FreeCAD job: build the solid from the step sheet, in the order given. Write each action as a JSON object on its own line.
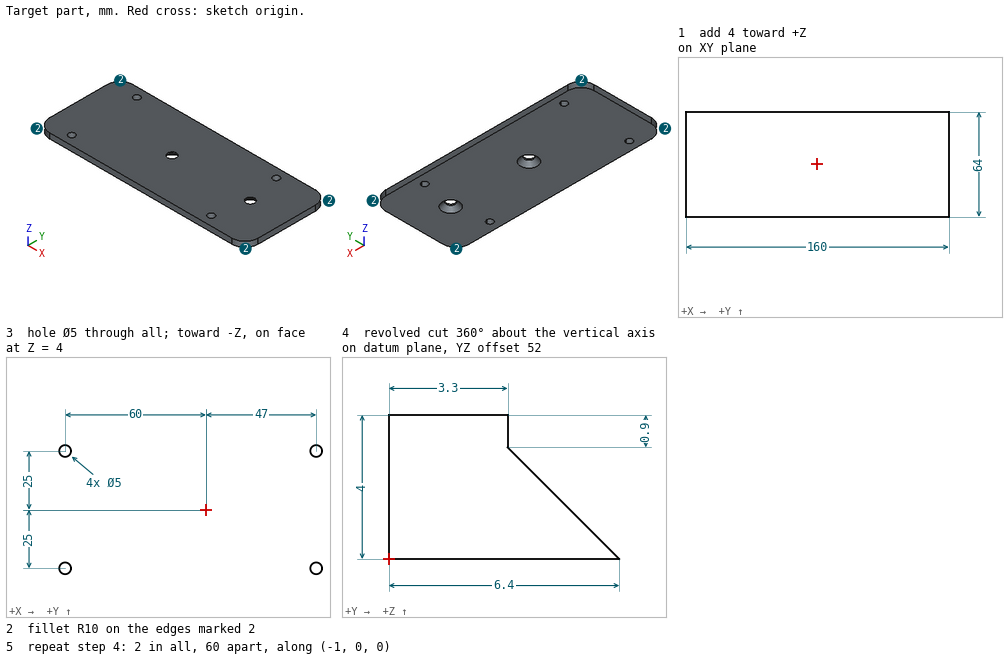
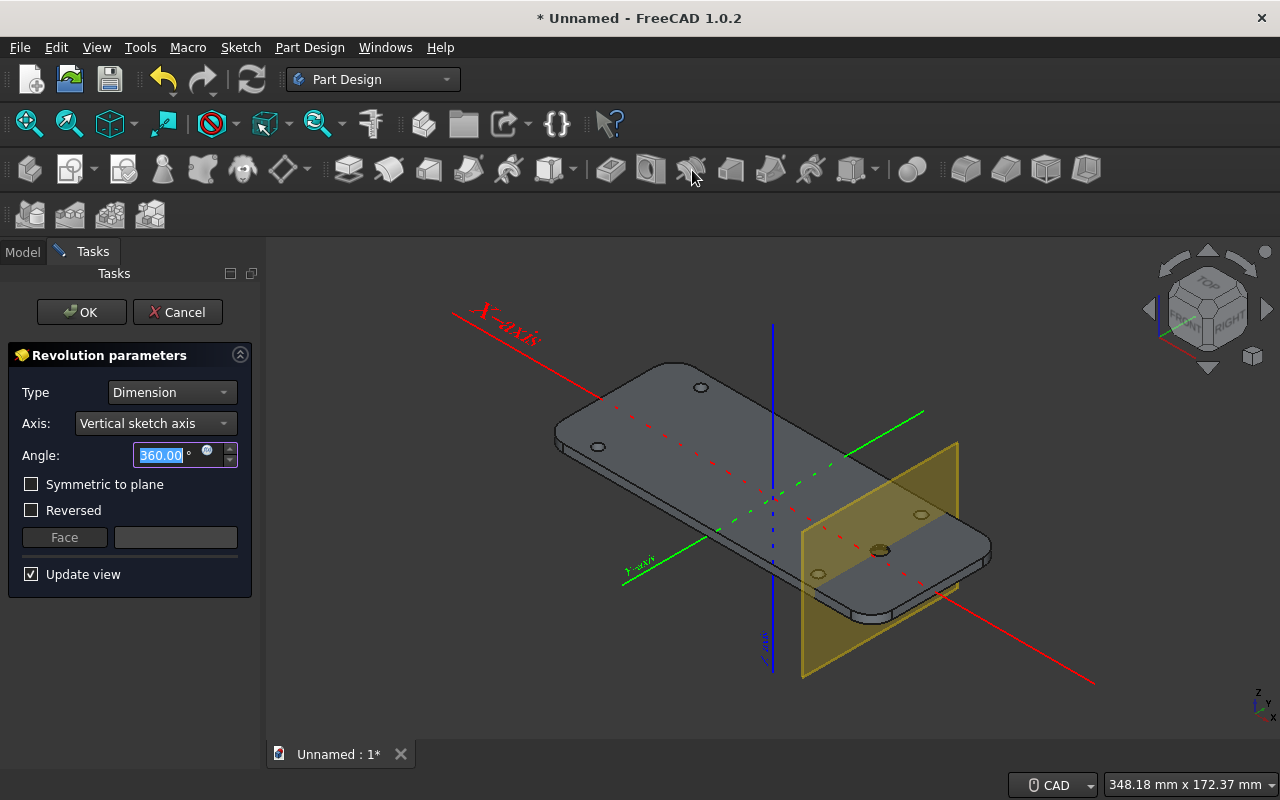
{"action": "left_click", "coordinate": [82, 312]}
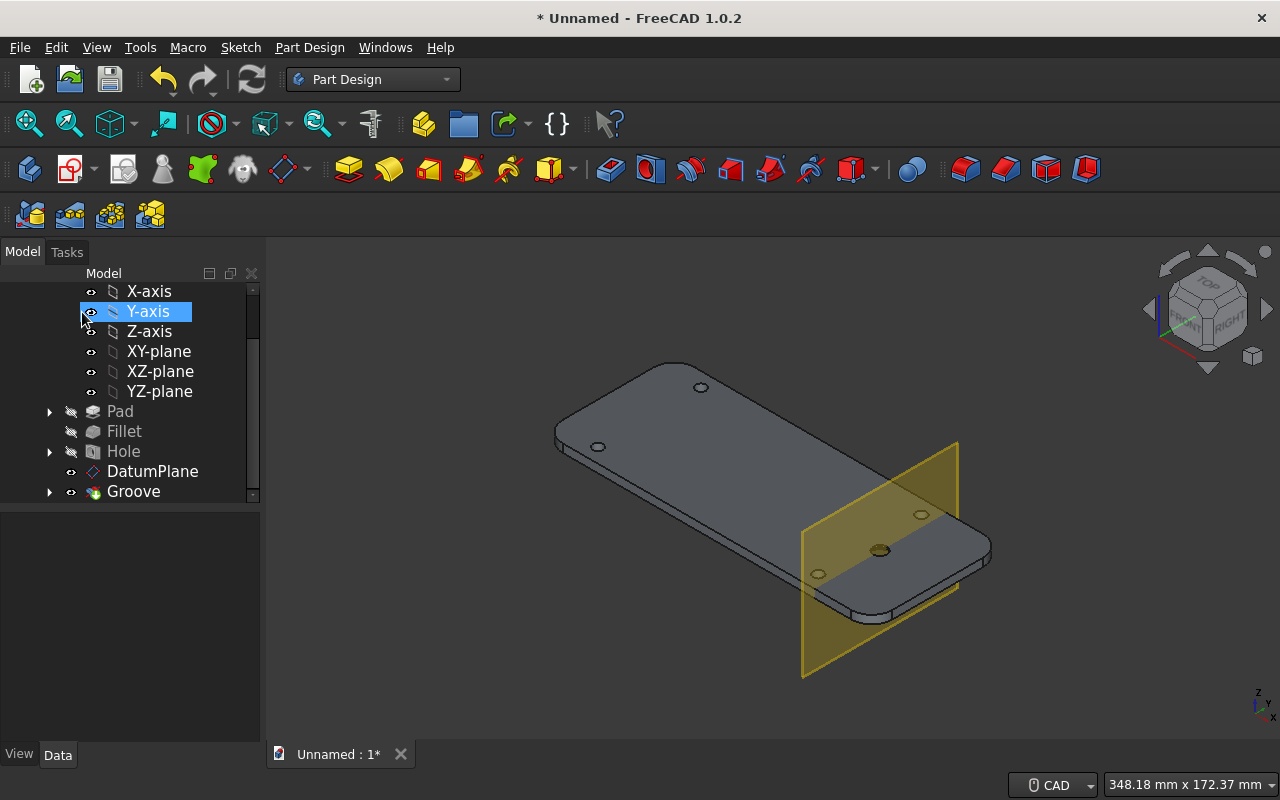
{"action": "left_click", "coordinate": [116, 472]}
{"action": "key", "text": "space"}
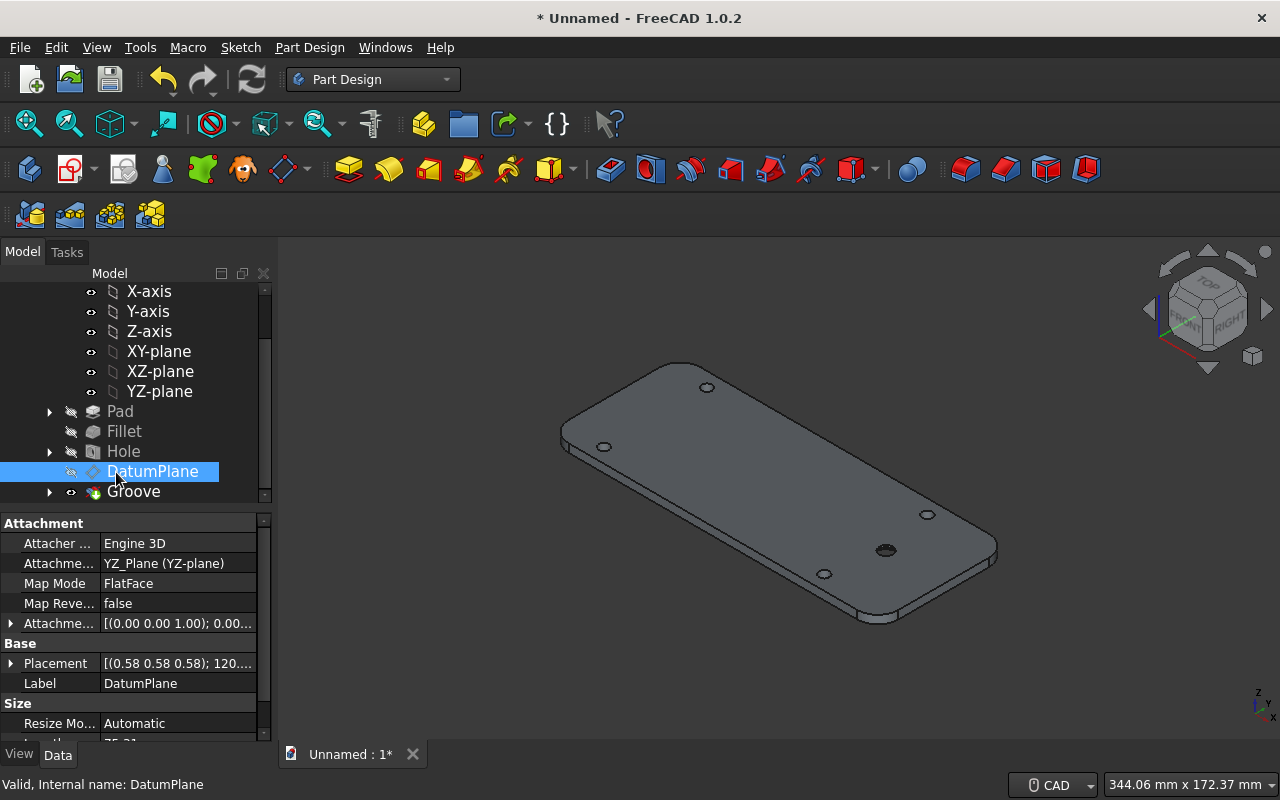
{"action": "left_click", "coordinate": [116, 492]}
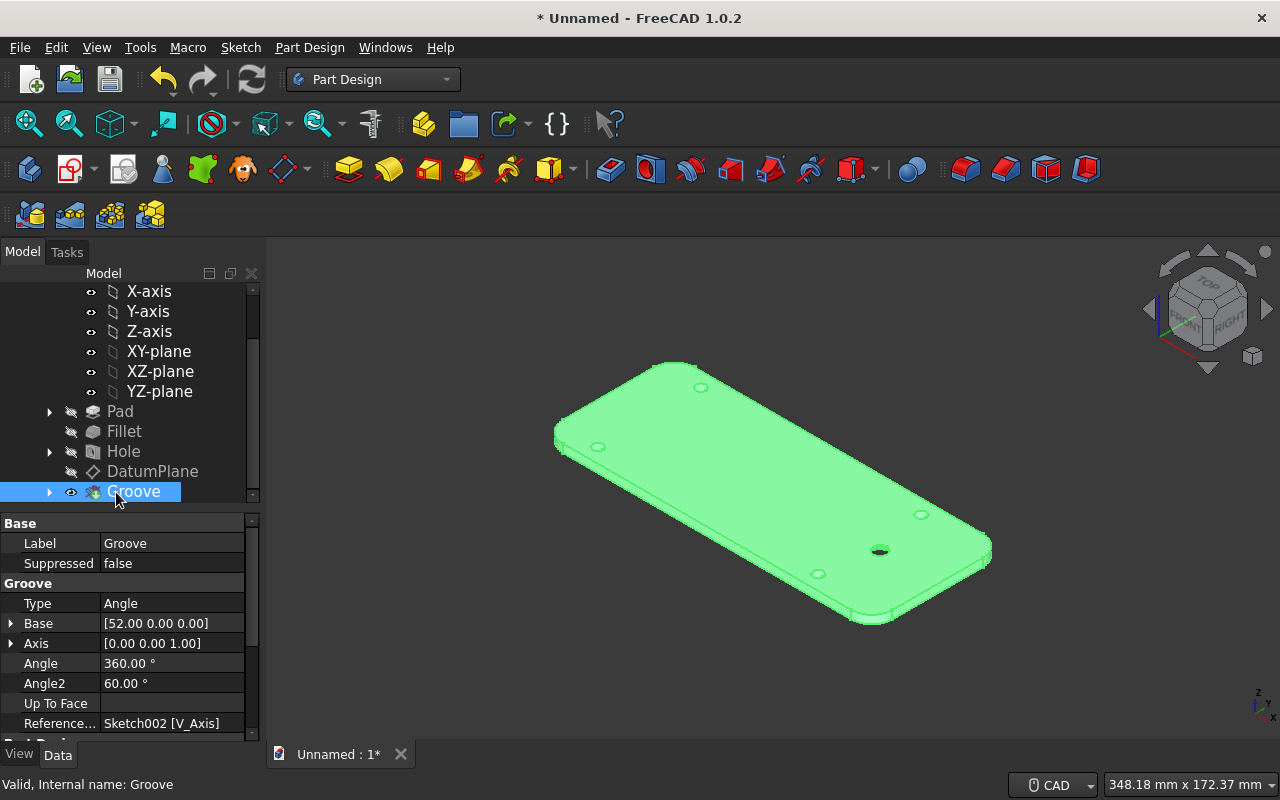
{"action": "left_click", "coordinate": [70, 214]}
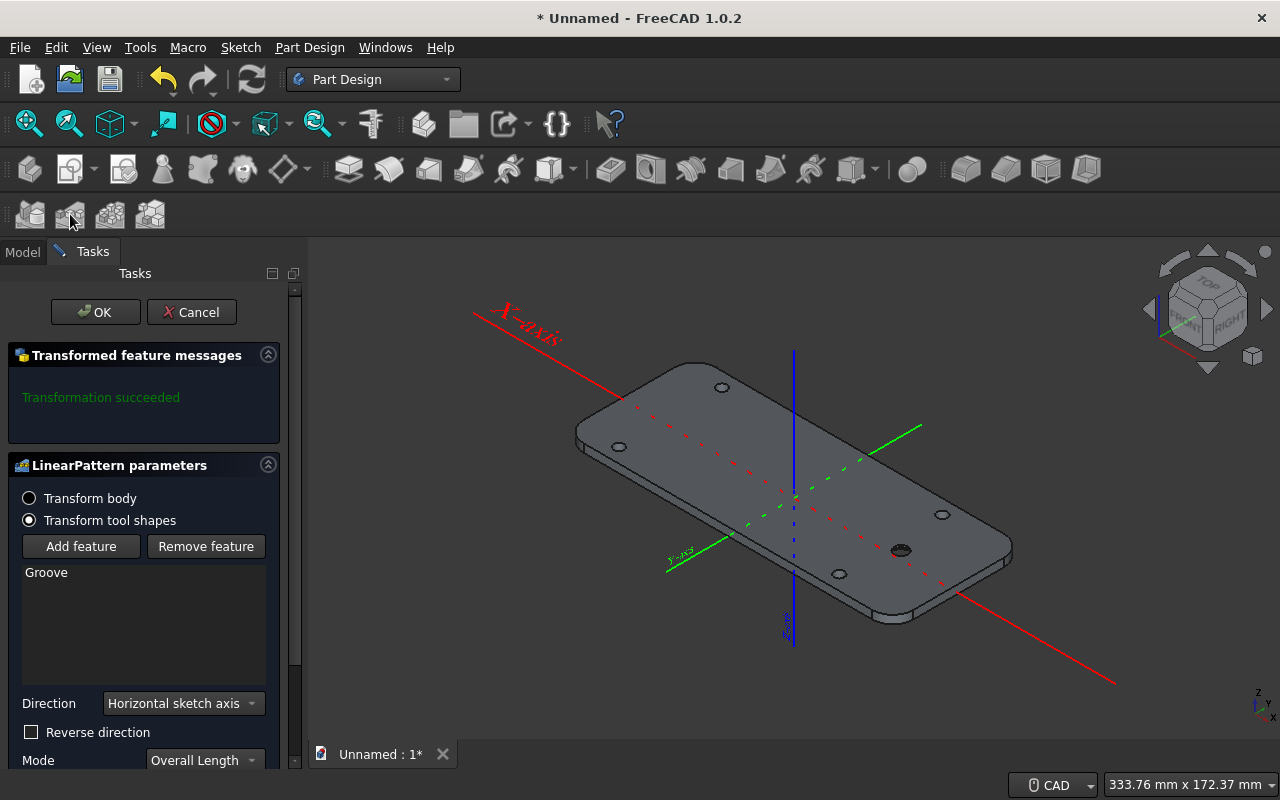
{"action": "left_click", "coordinate": [184, 704]}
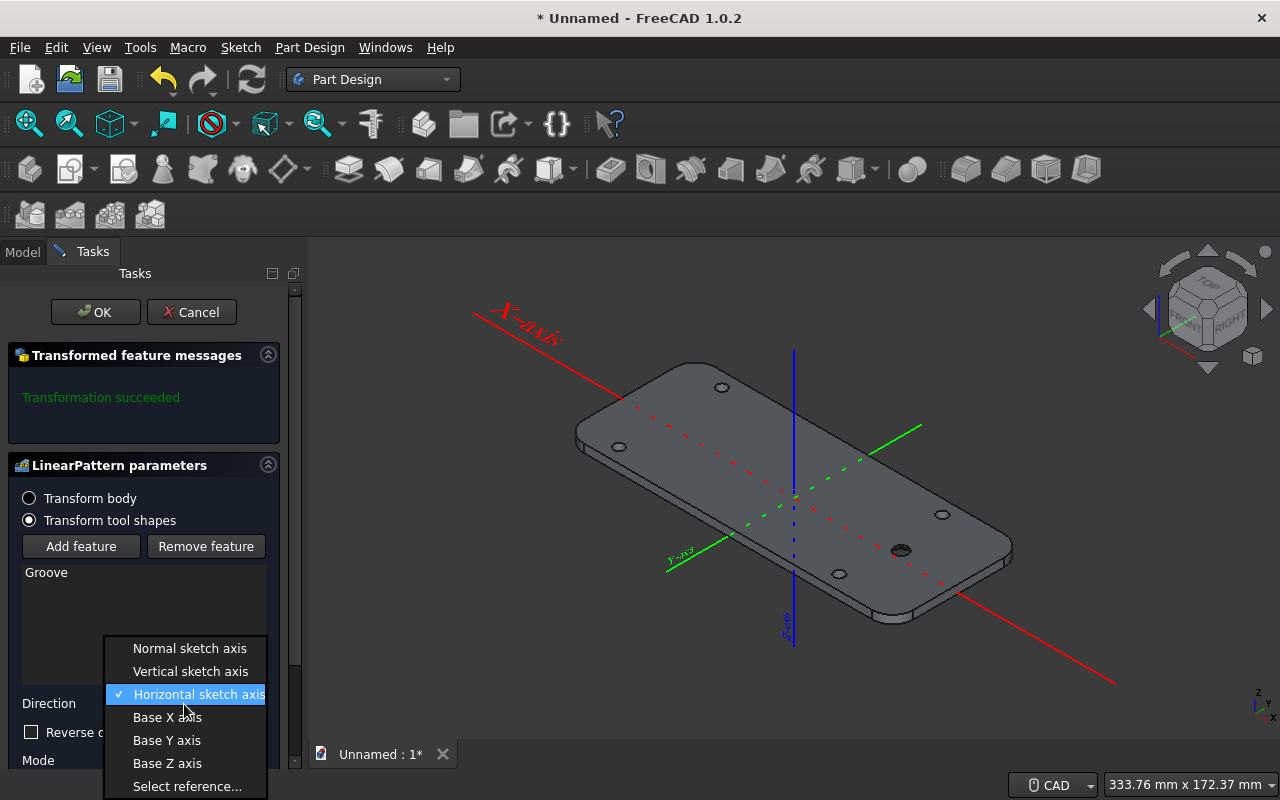
{"action": "left_click", "coordinate": [184, 718]}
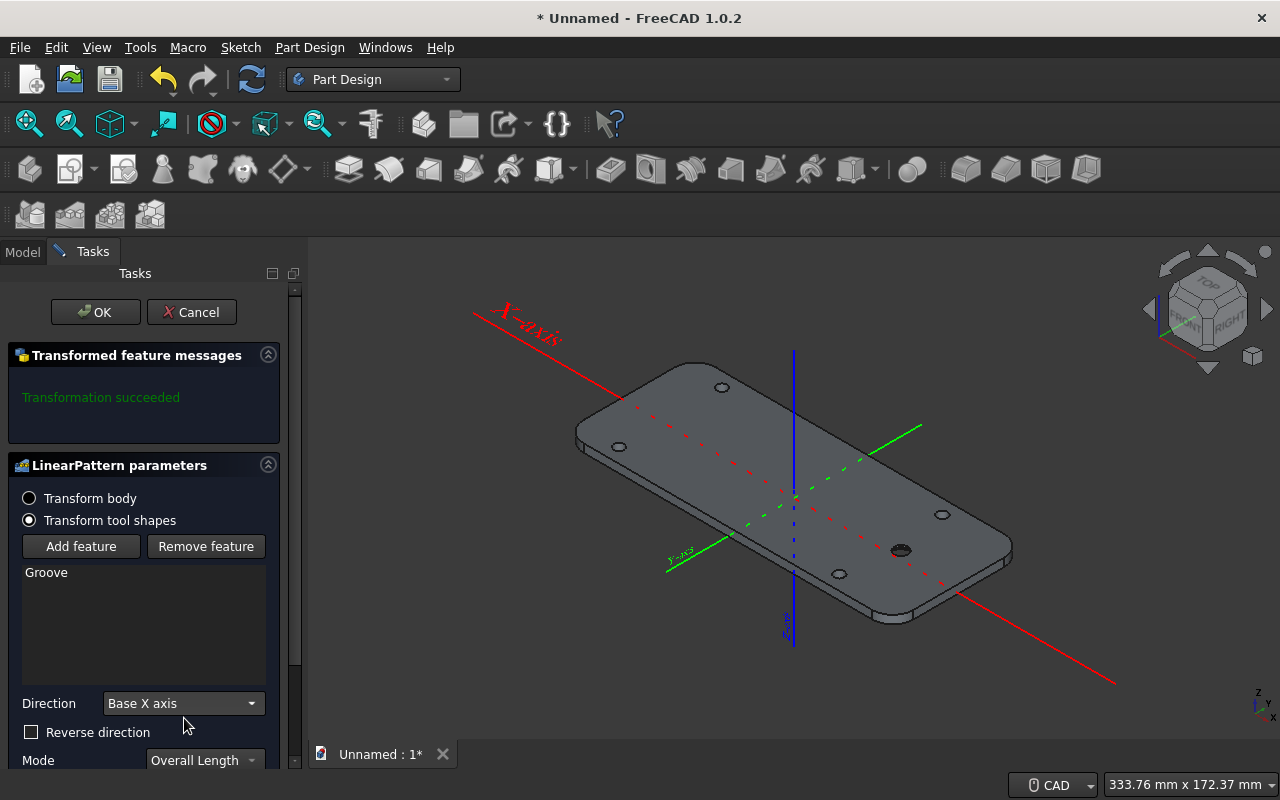
{"action": "scroll", "coordinate": [295, 526], "scroll_direction": "down", "scroll_amount": 2}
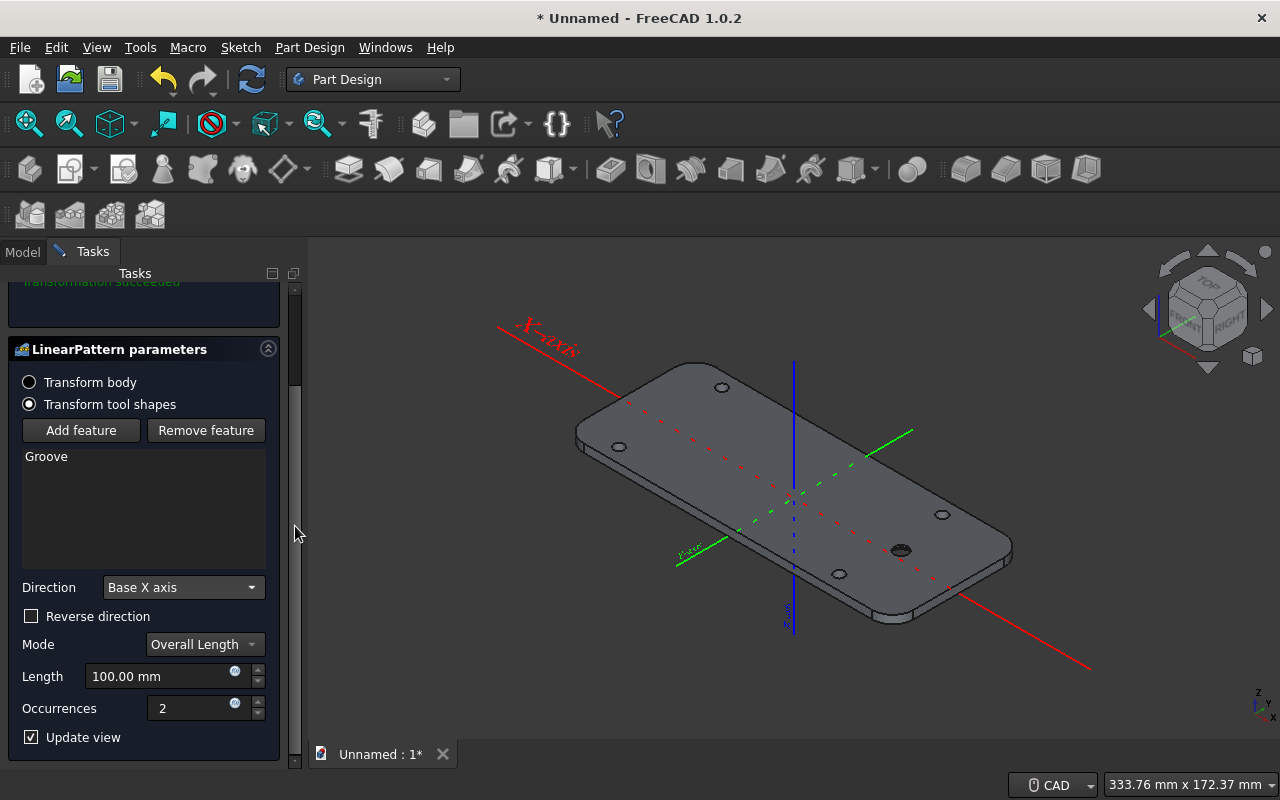
{"action": "left_click", "coordinate": [206, 644]}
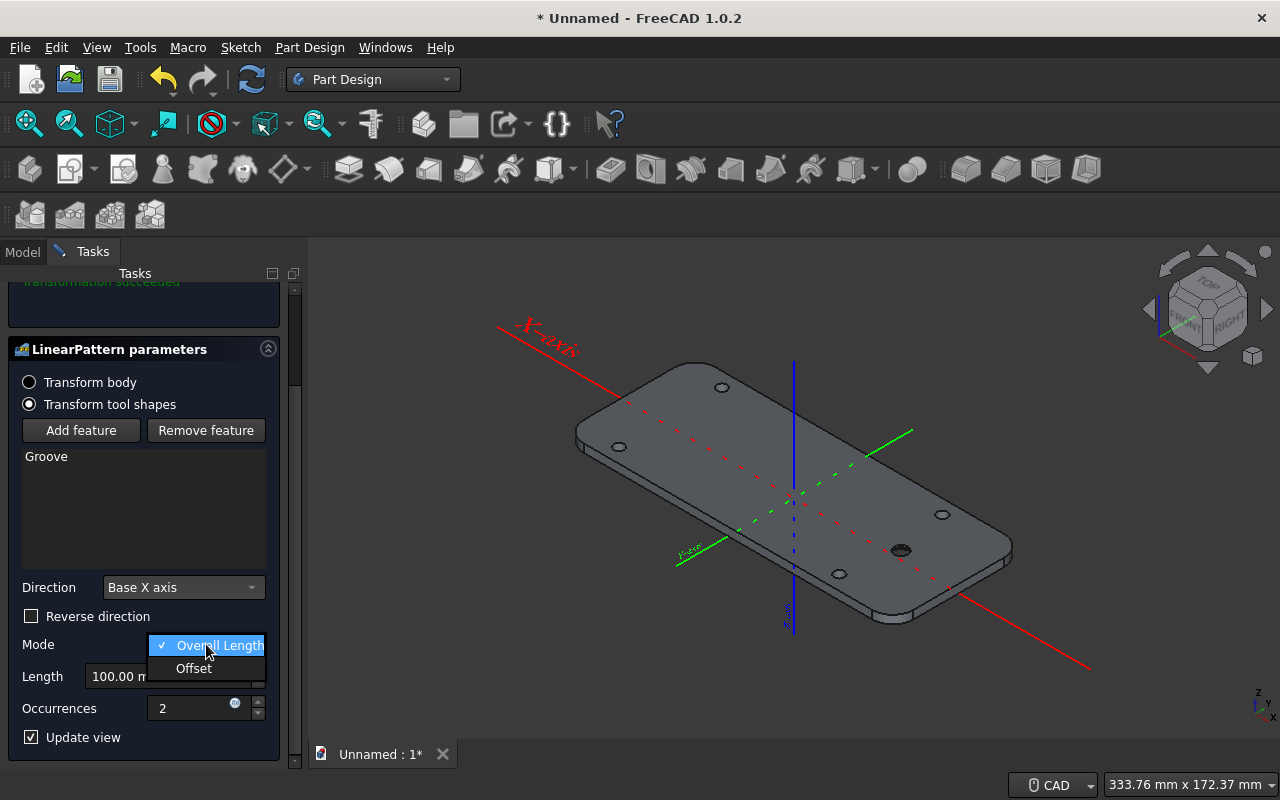
{"action": "left_click", "coordinate": [206, 668]}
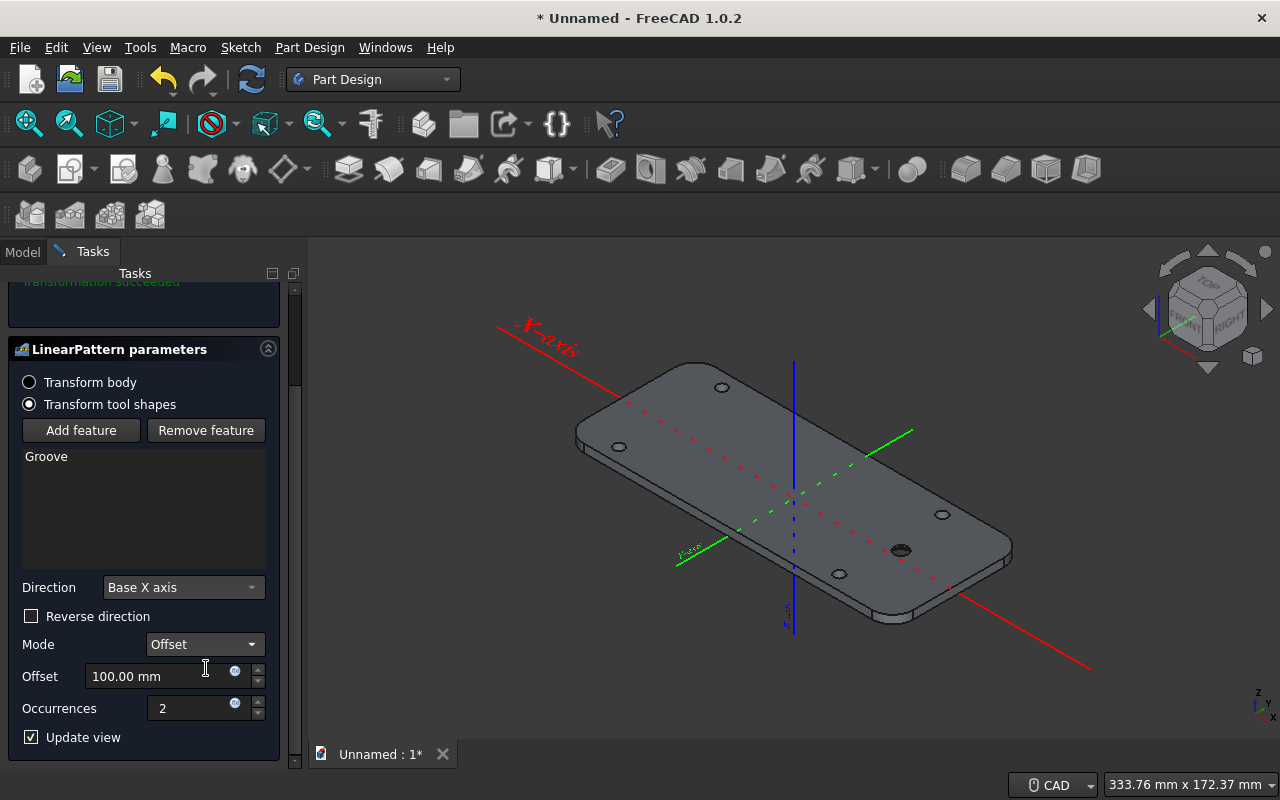
{"action": "triple_click", "coordinate": [168, 676]}